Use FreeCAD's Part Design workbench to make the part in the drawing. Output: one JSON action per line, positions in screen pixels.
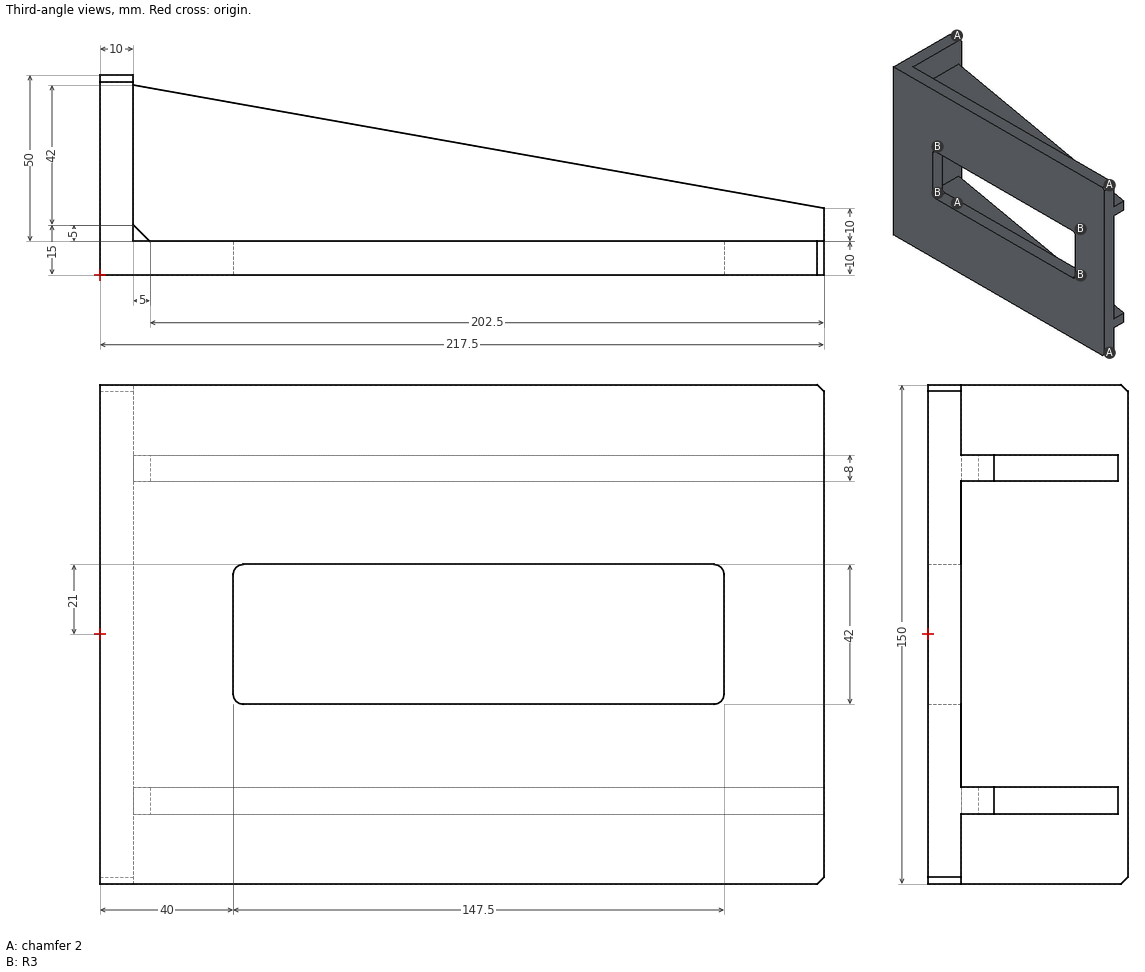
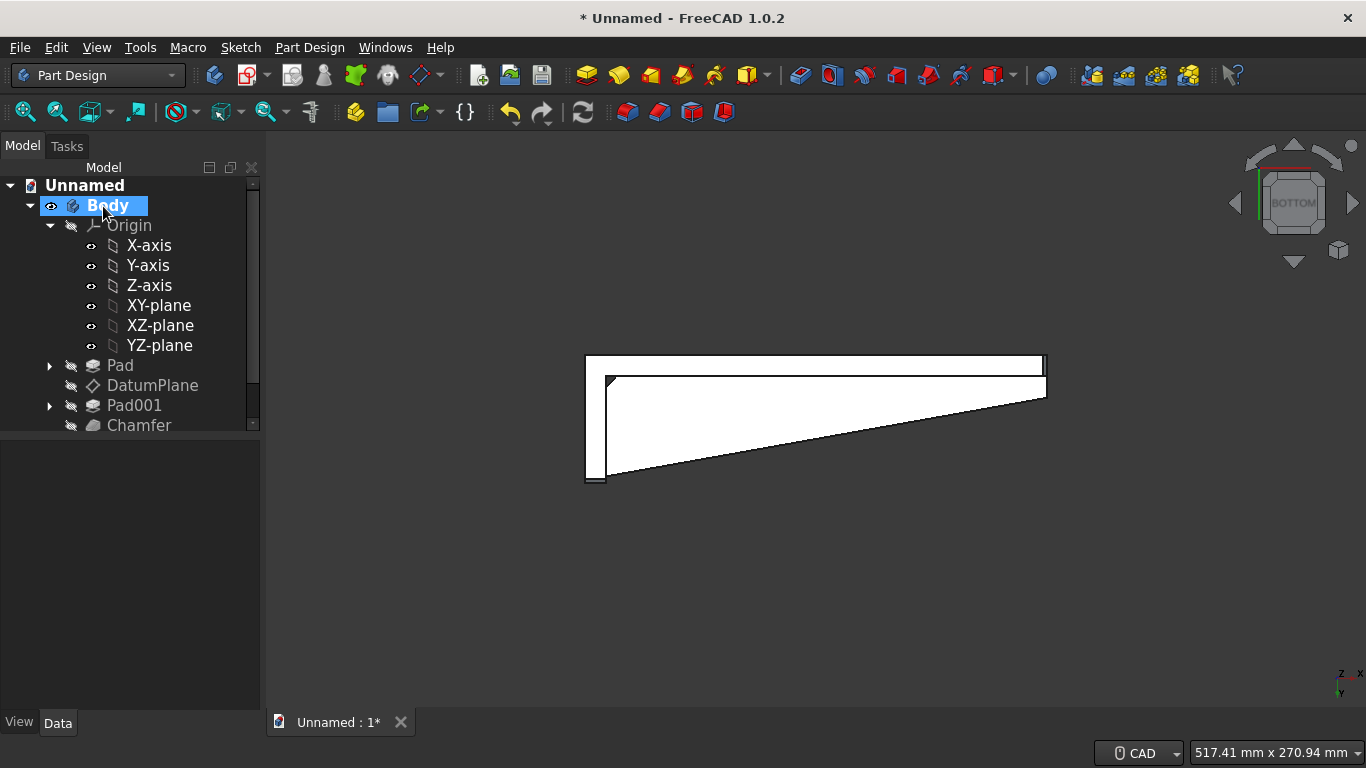
{"action": "left_click", "coordinate": [26, 112]}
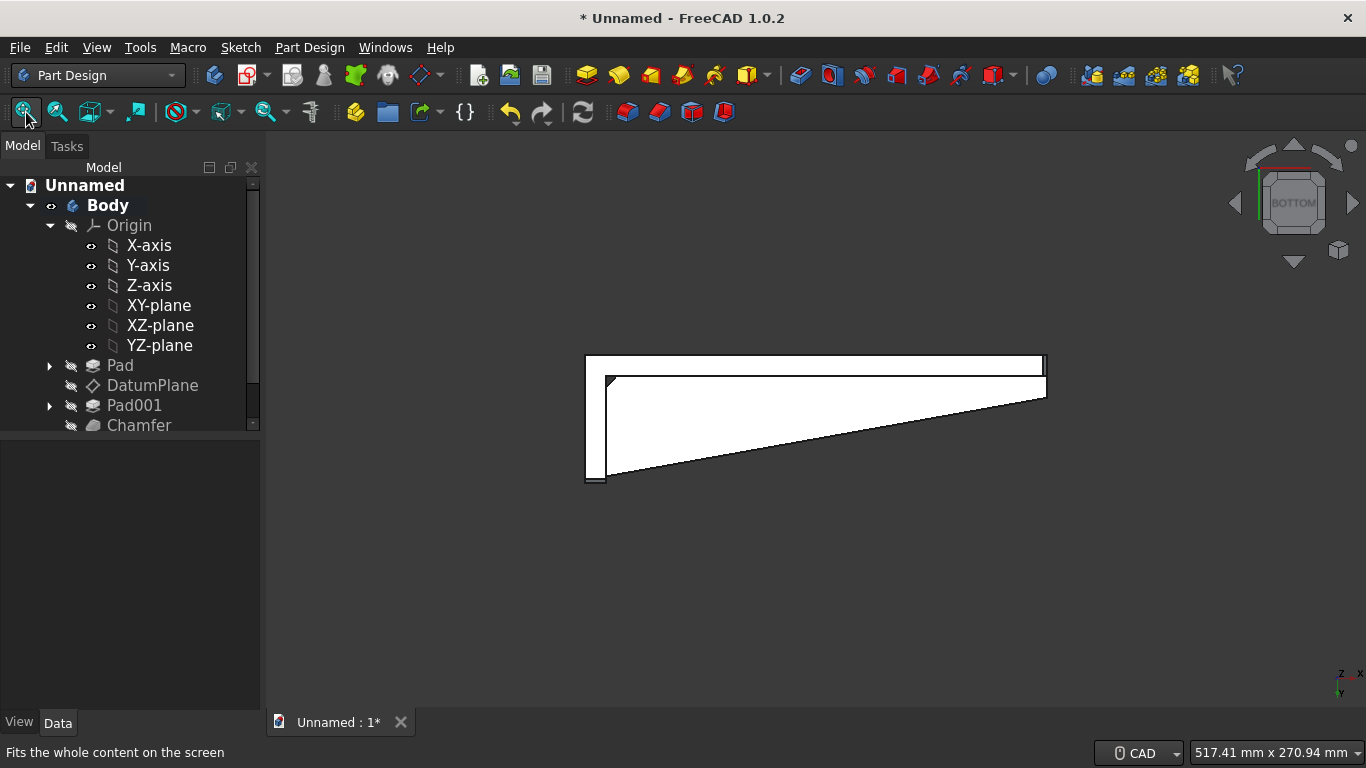
{"action": "key", "text": "4"}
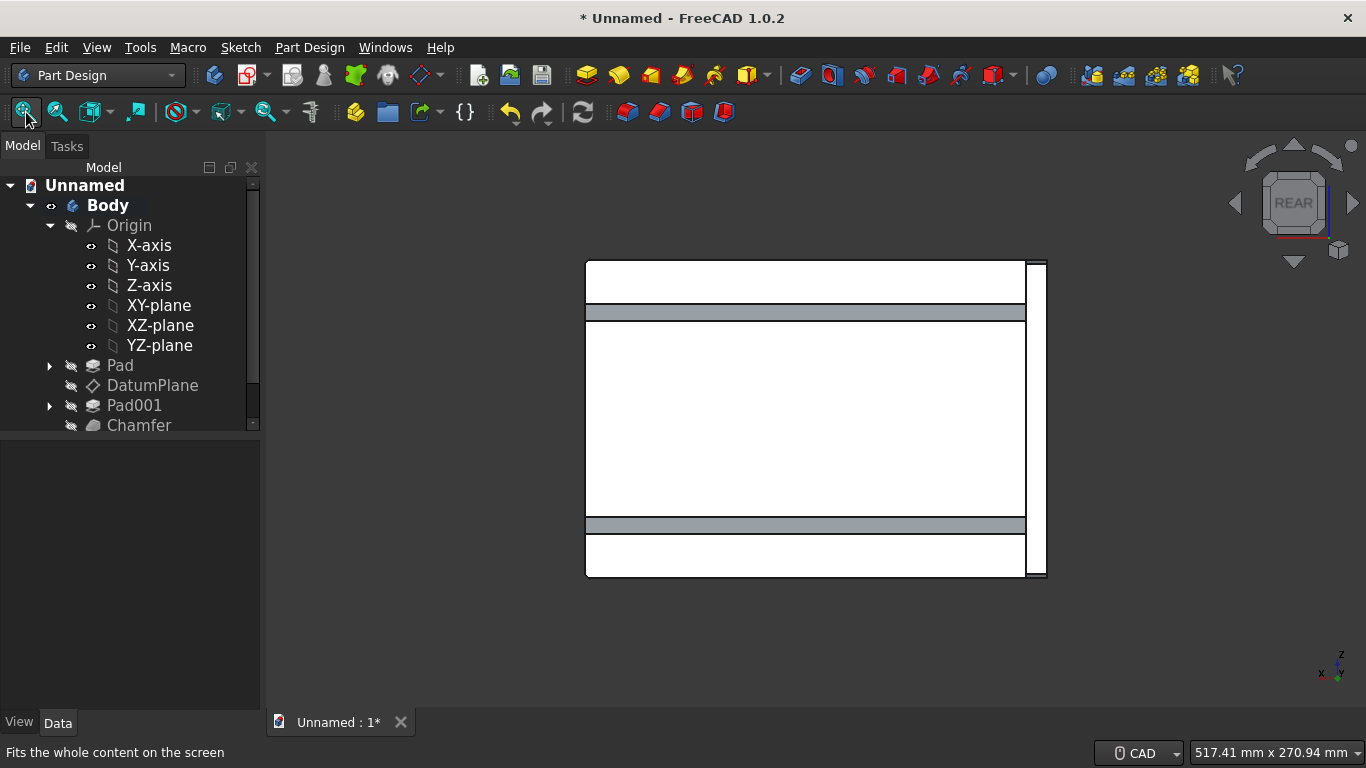
{"action": "left_click", "coordinate": [742, 418]}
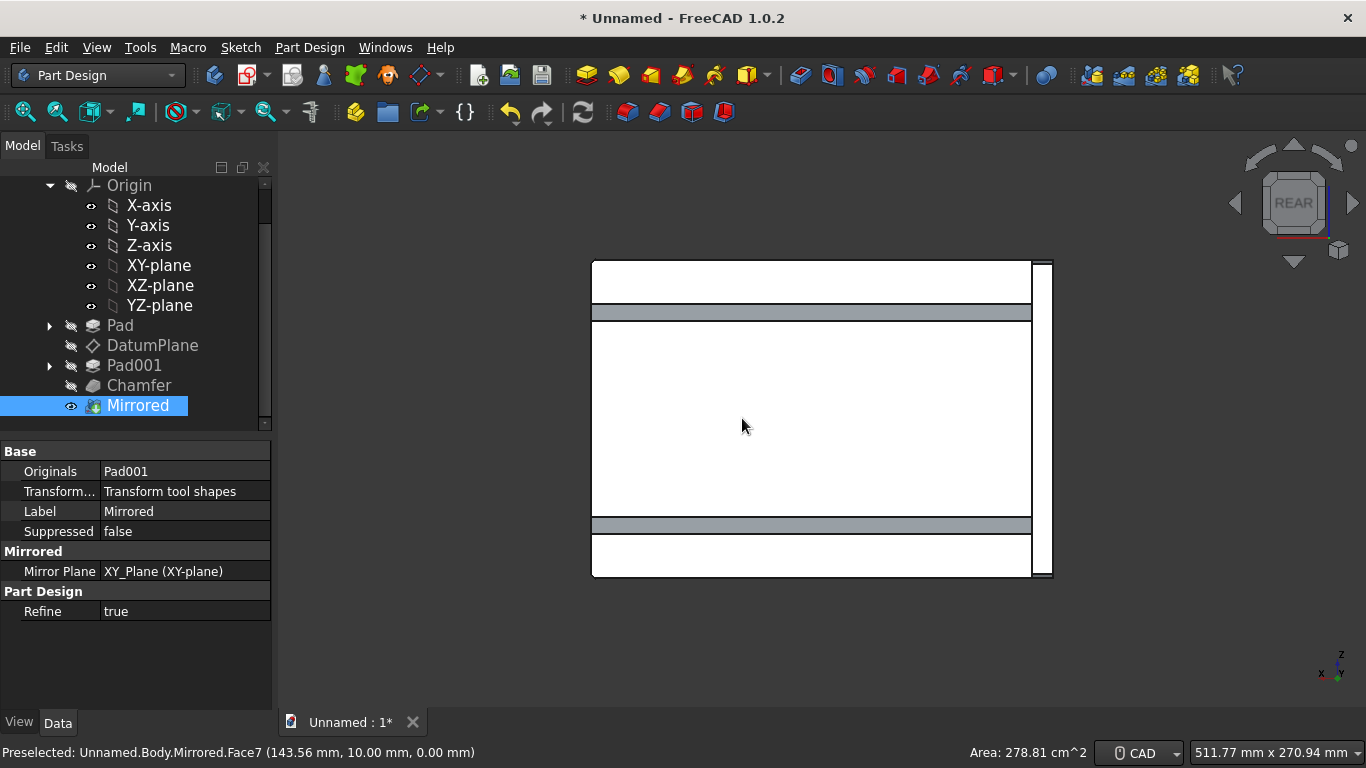
{"action": "left_click", "coordinate": [248, 76]}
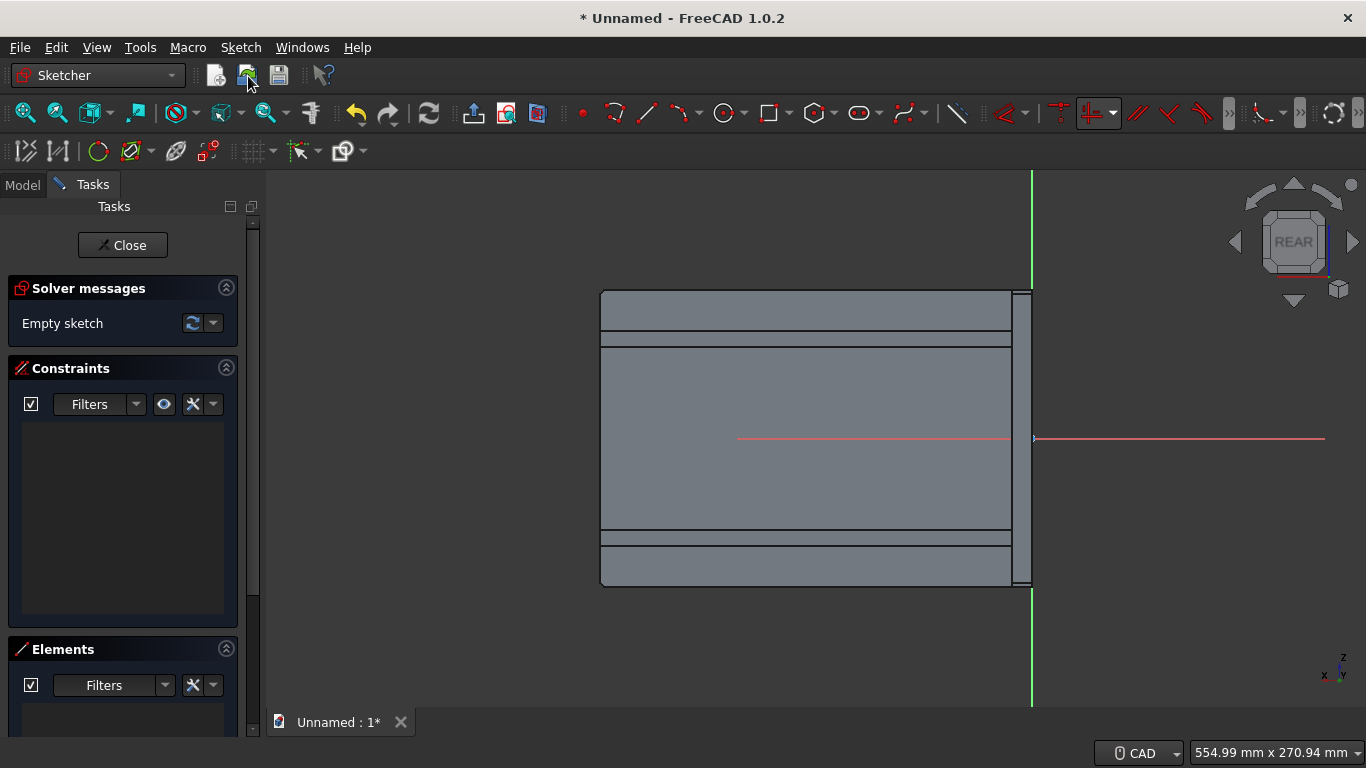
{"action": "left_click", "coordinate": [538, 114]}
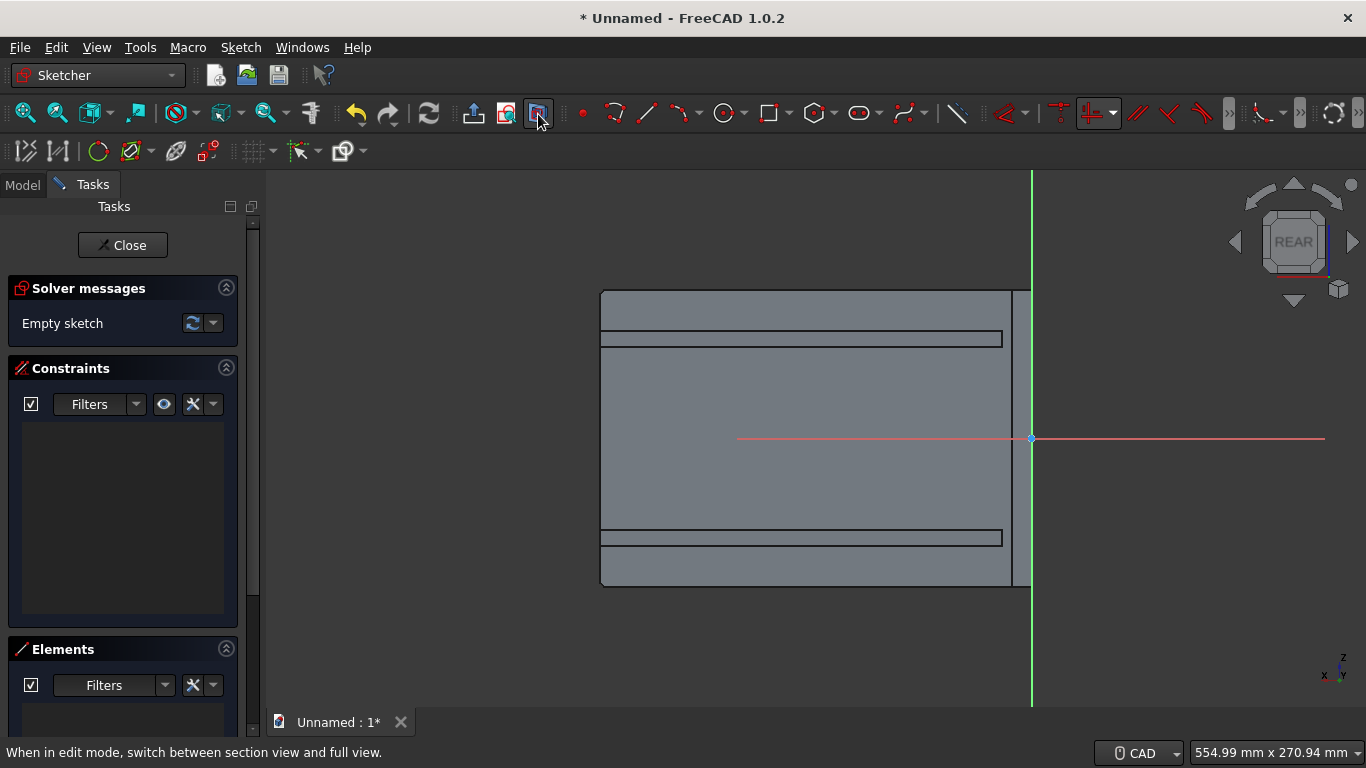
{"action": "scroll", "coordinate": [965, 438], "scroll_direction": "up", "scroll_amount": 3}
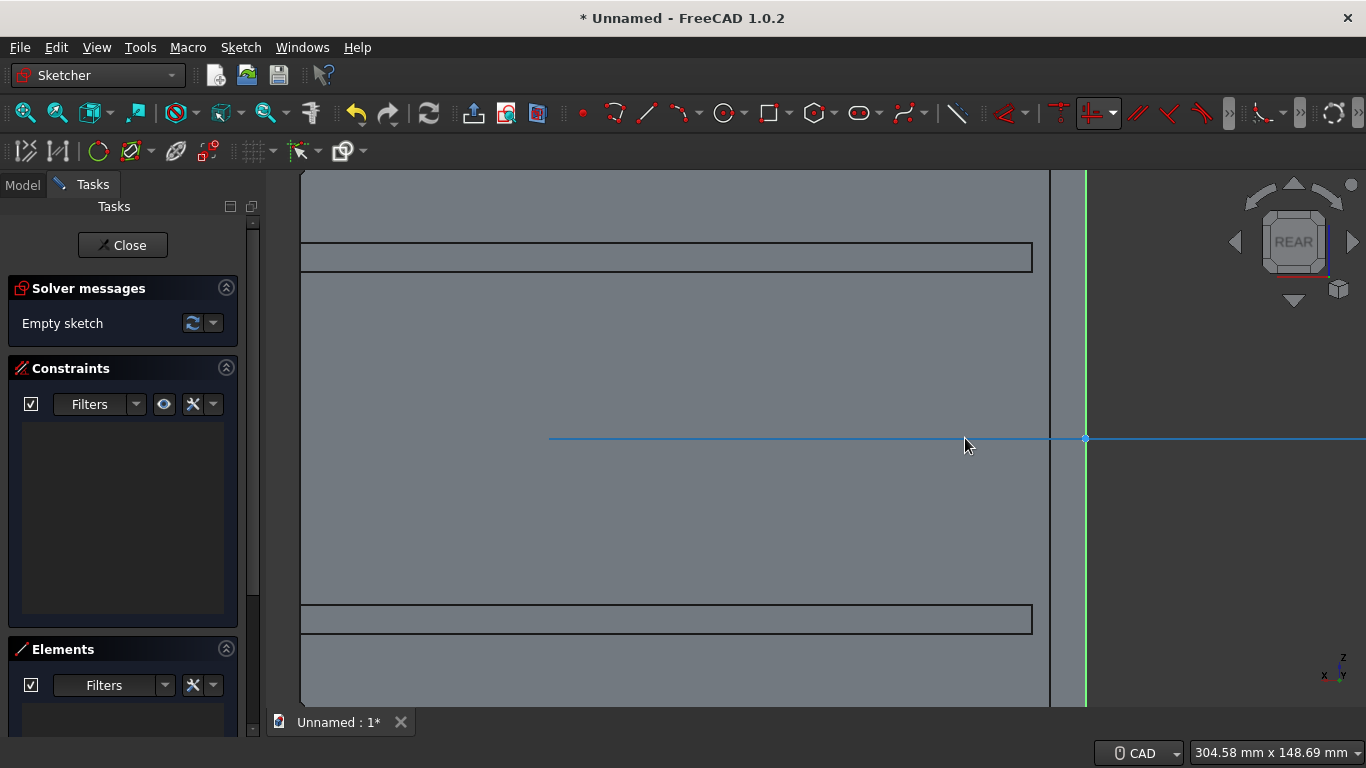
{"action": "left_click", "coordinate": [770, 114]}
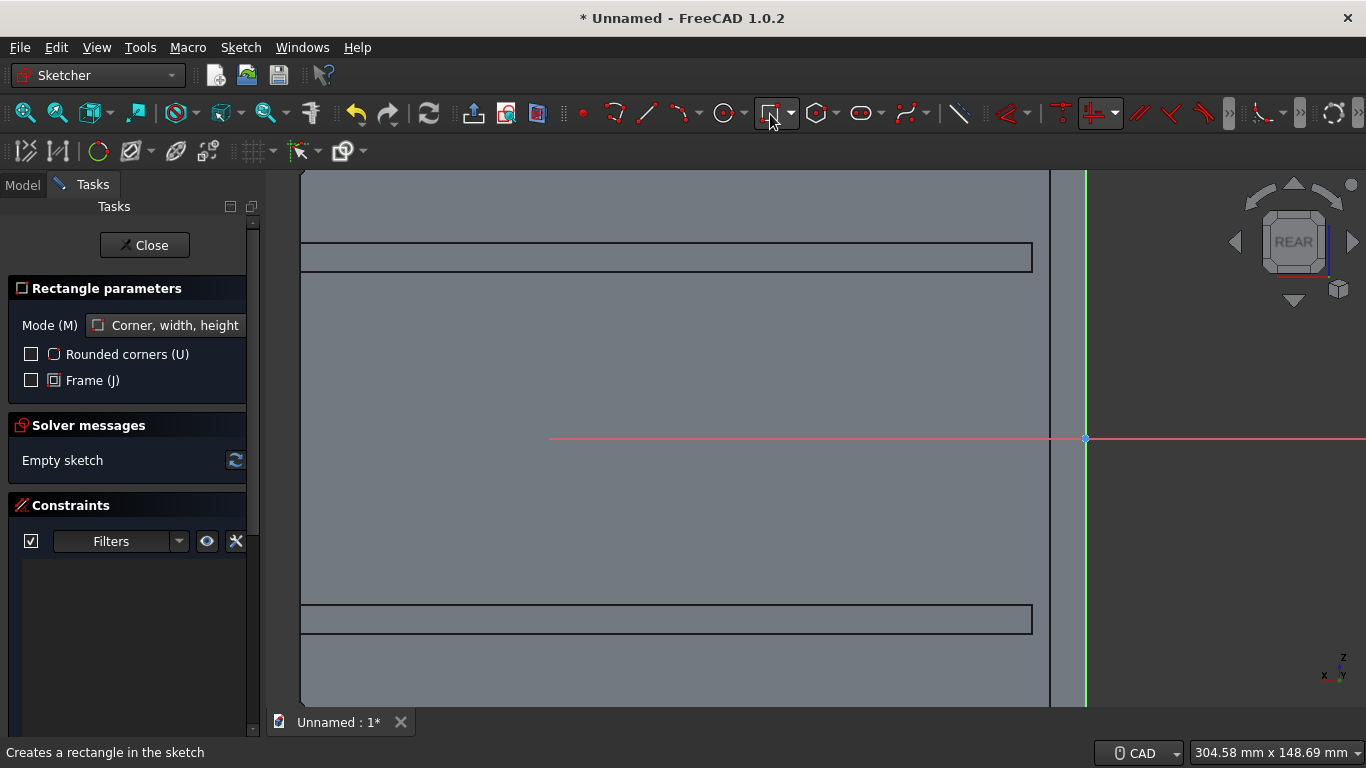
{"action": "left_click", "coordinate": [409, 363]}
{"action": "left_click", "coordinate": [941, 514]}
{"action": "key", "text": "Escape"}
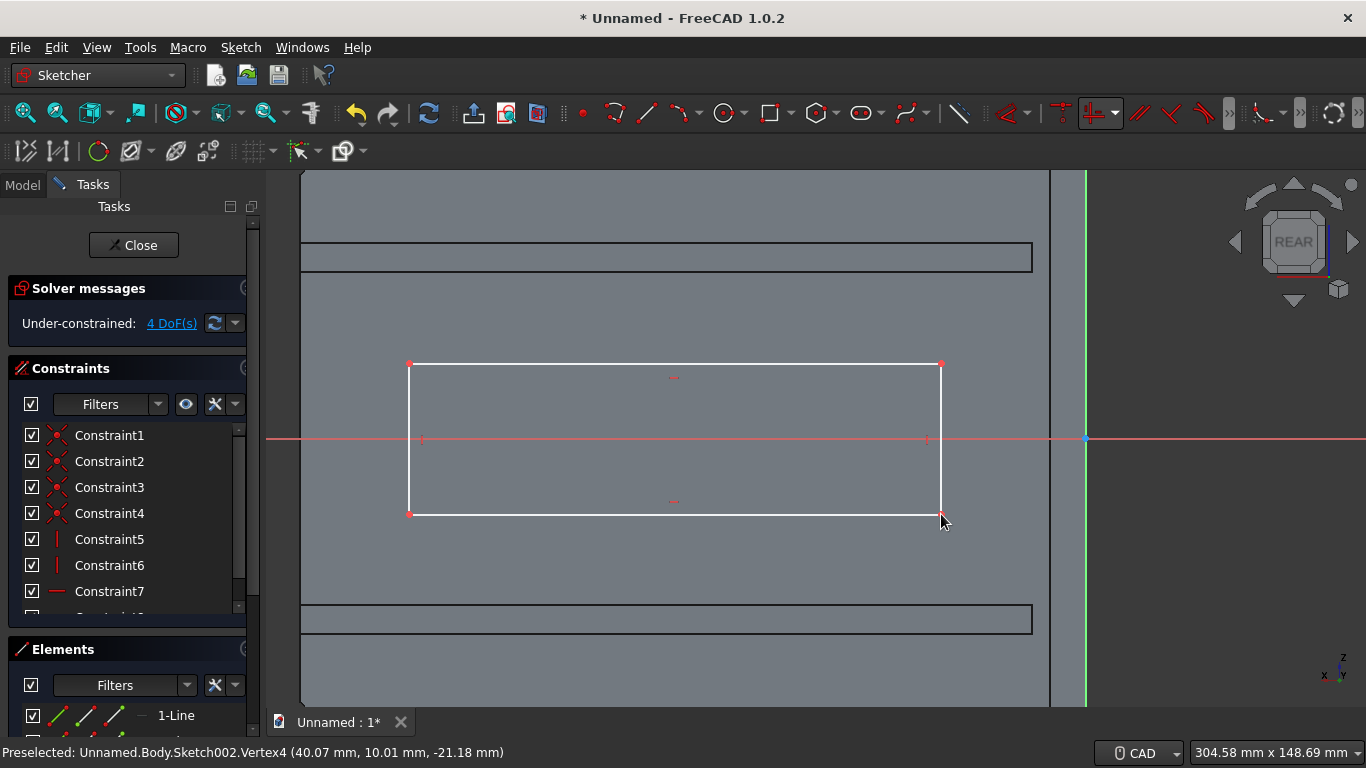
{"action": "left_click", "coordinate": [1006, 114]}